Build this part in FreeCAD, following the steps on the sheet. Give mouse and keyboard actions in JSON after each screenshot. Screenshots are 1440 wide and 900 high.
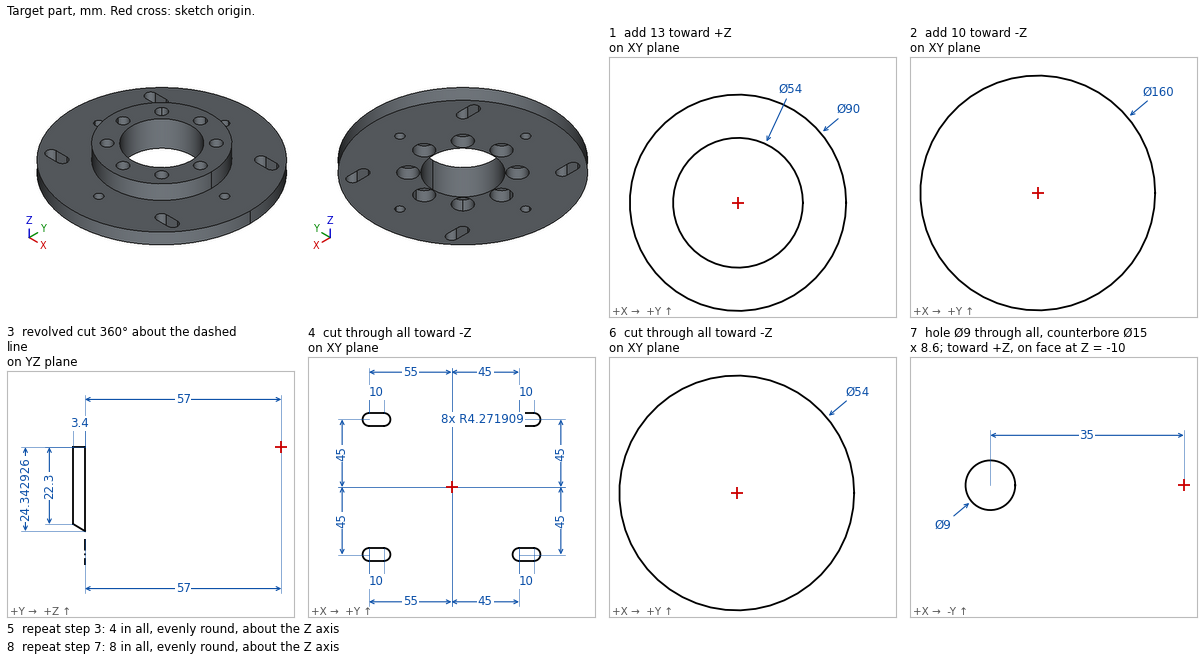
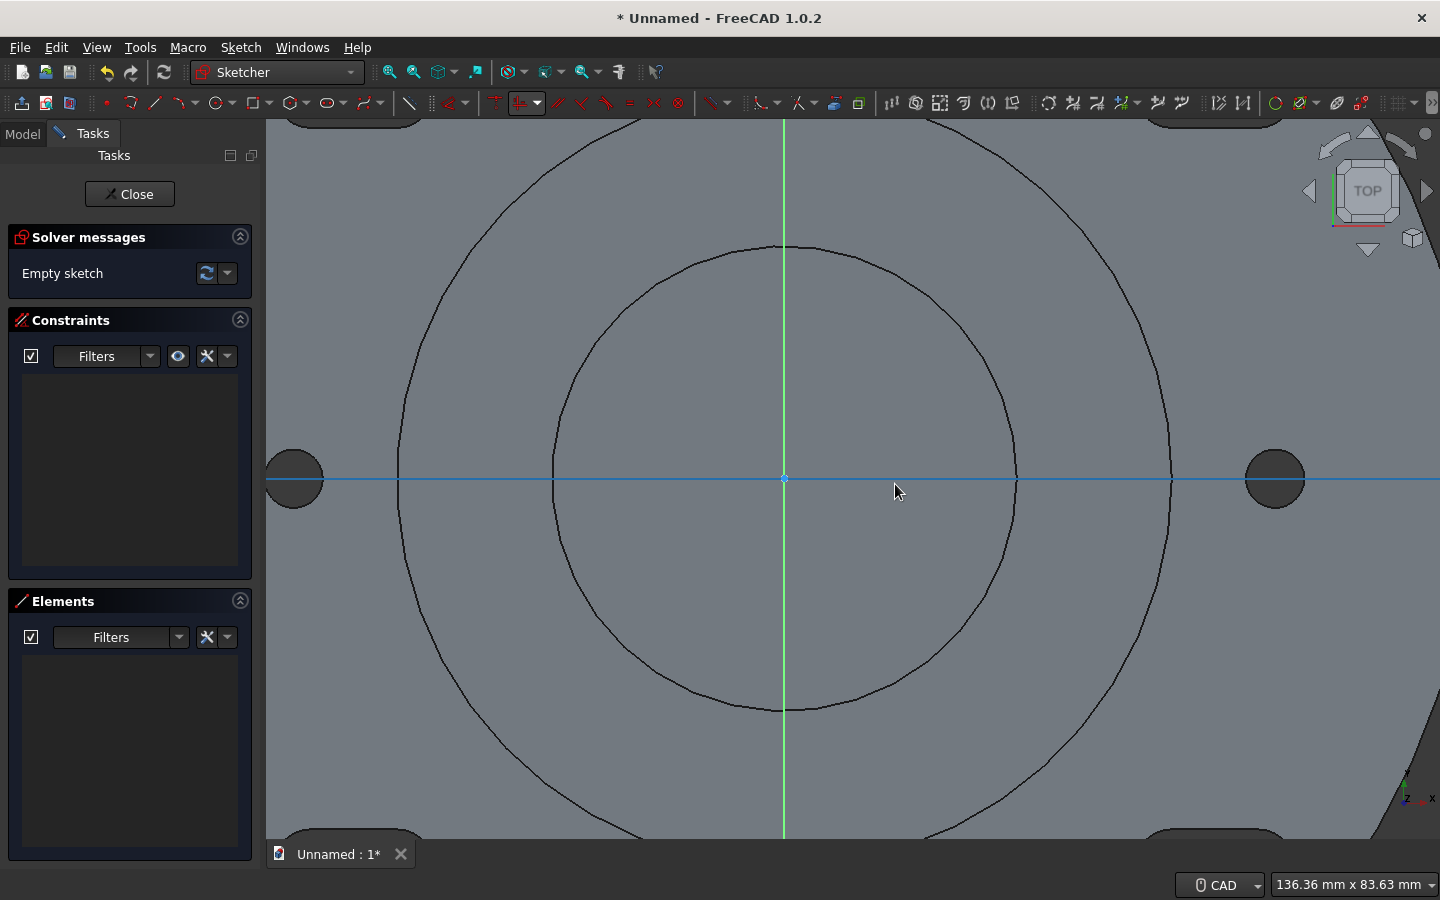
{"action": "key", "text": "g c"}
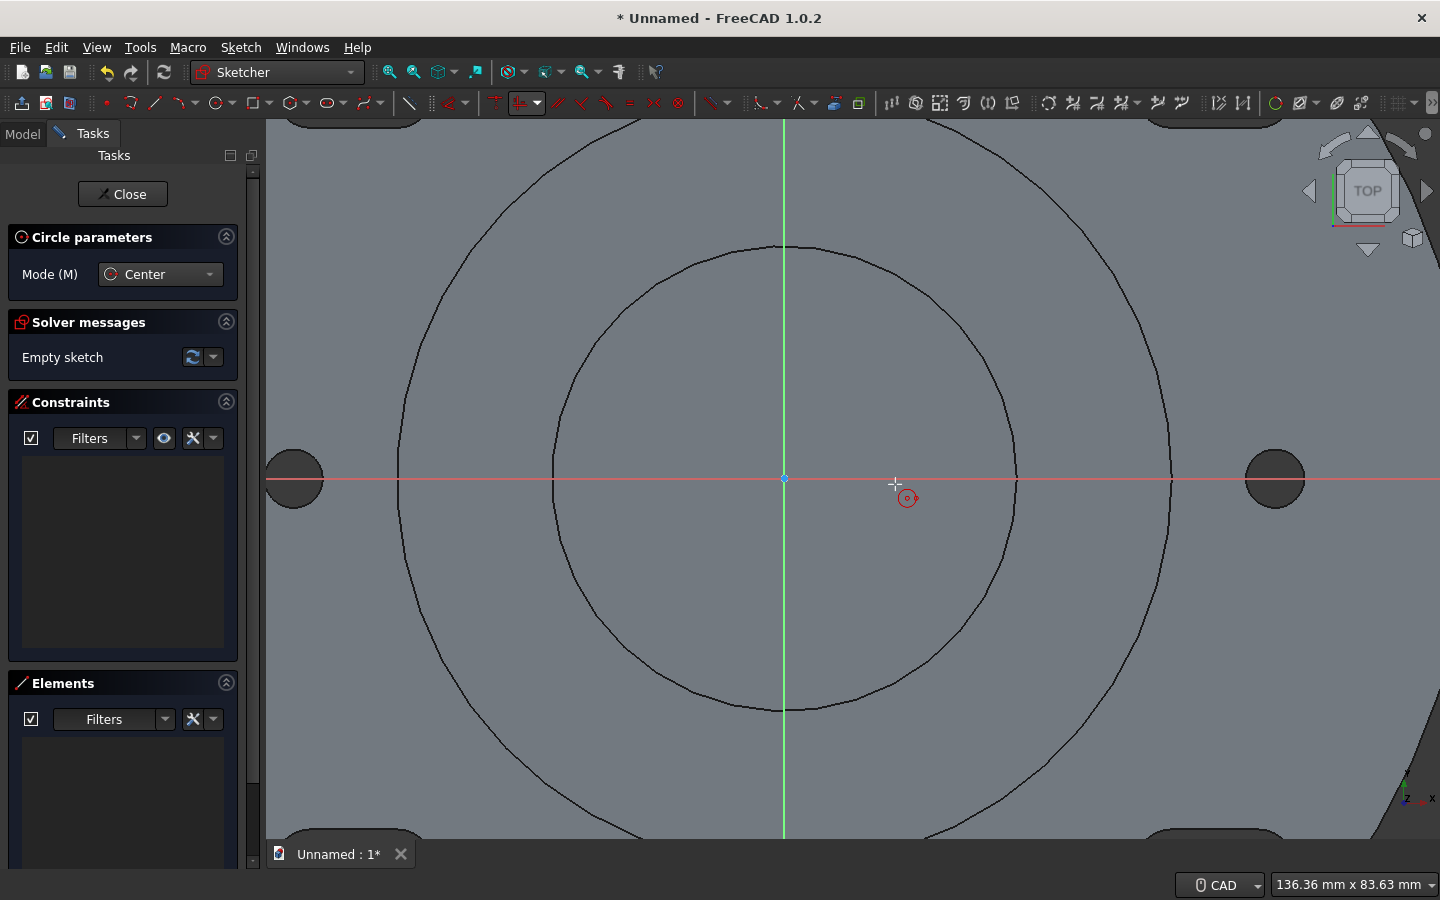
{"action": "left_click", "coordinate": [784, 479]}
{"action": "mouse_move", "coordinate": [949, 314]}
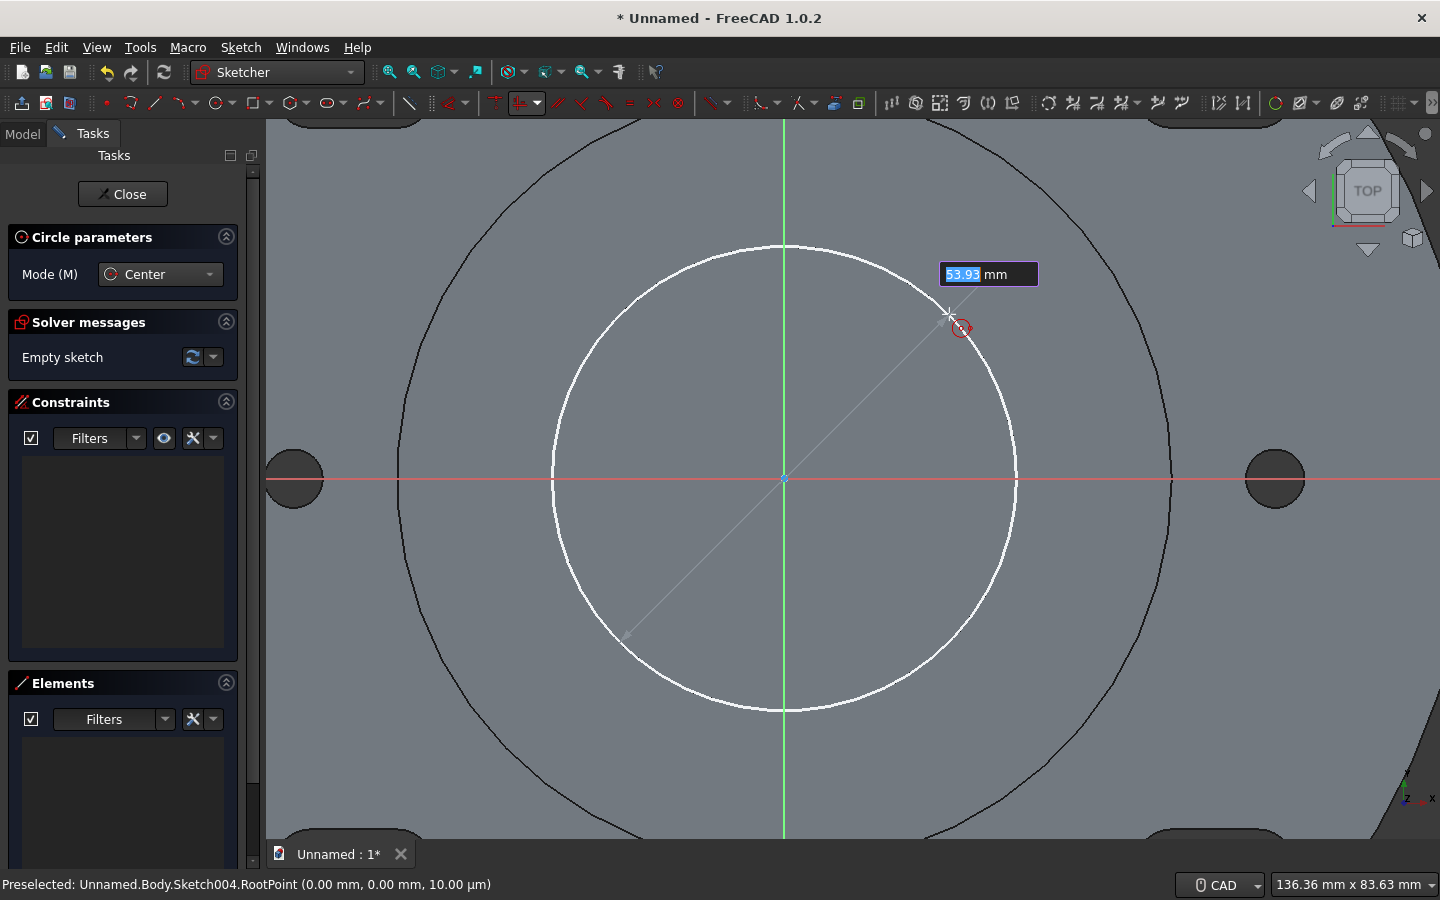
{"action": "type", "text": "54"}
{"action": "key", "text": "Return"}
{"action": "key", "text": "Escape"}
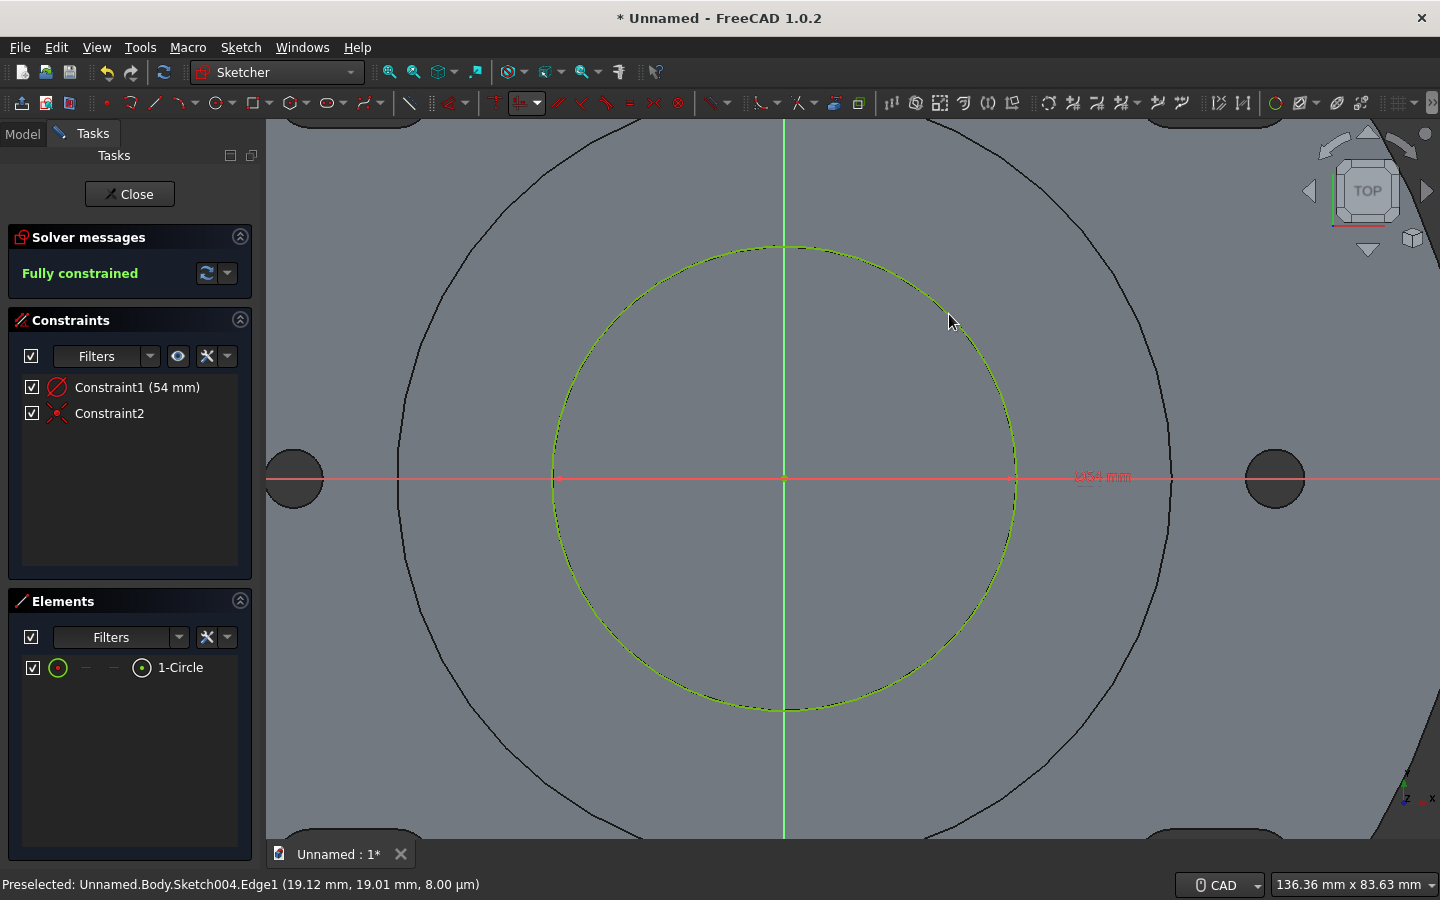
{"action": "left_click", "coordinate": [130, 194]}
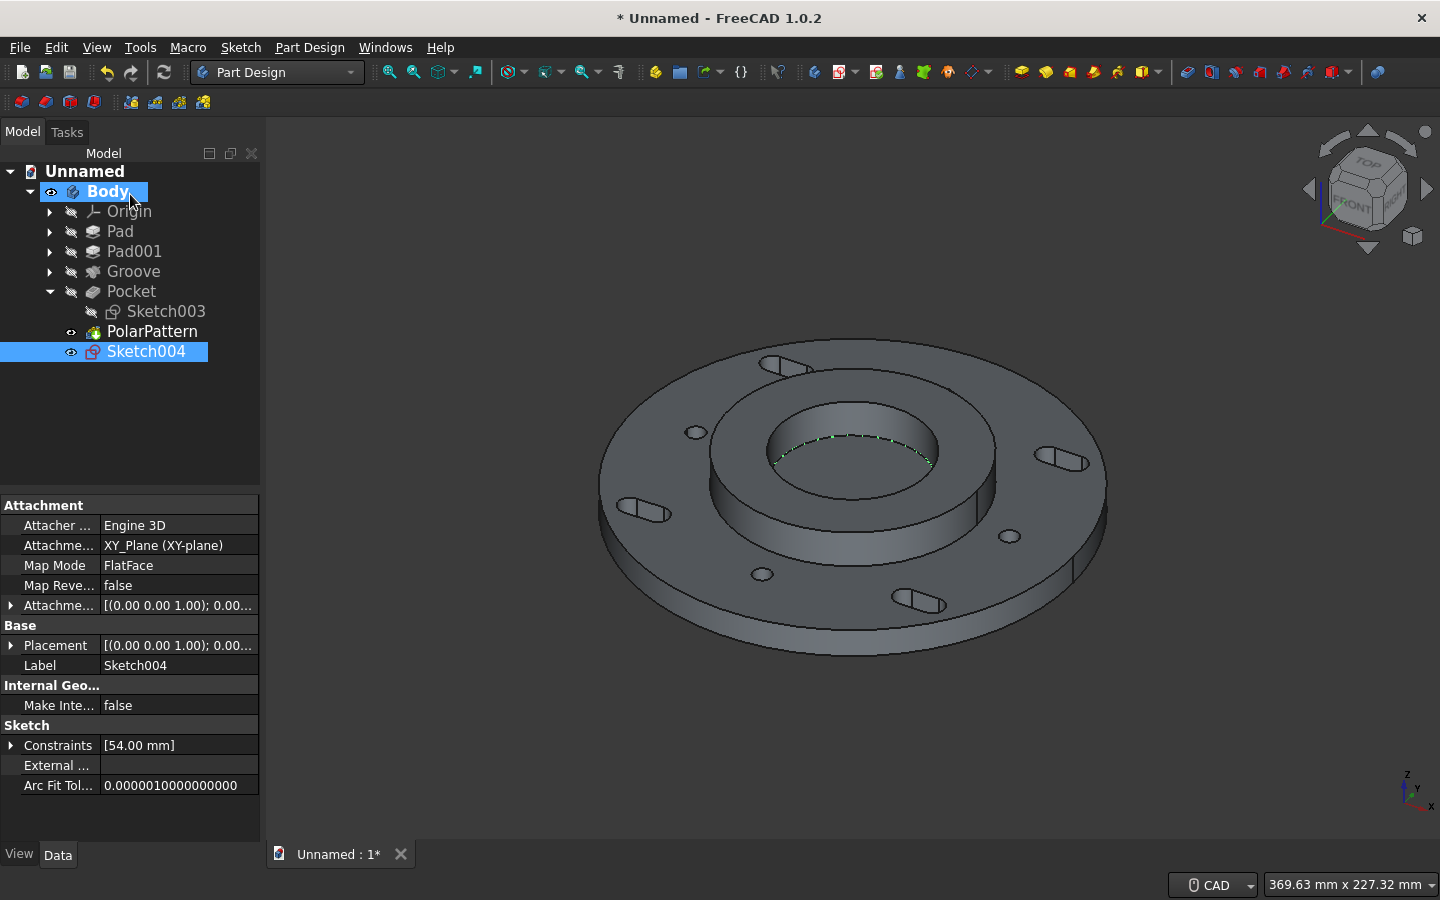
{"action": "left_click", "coordinate": [1188, 72]}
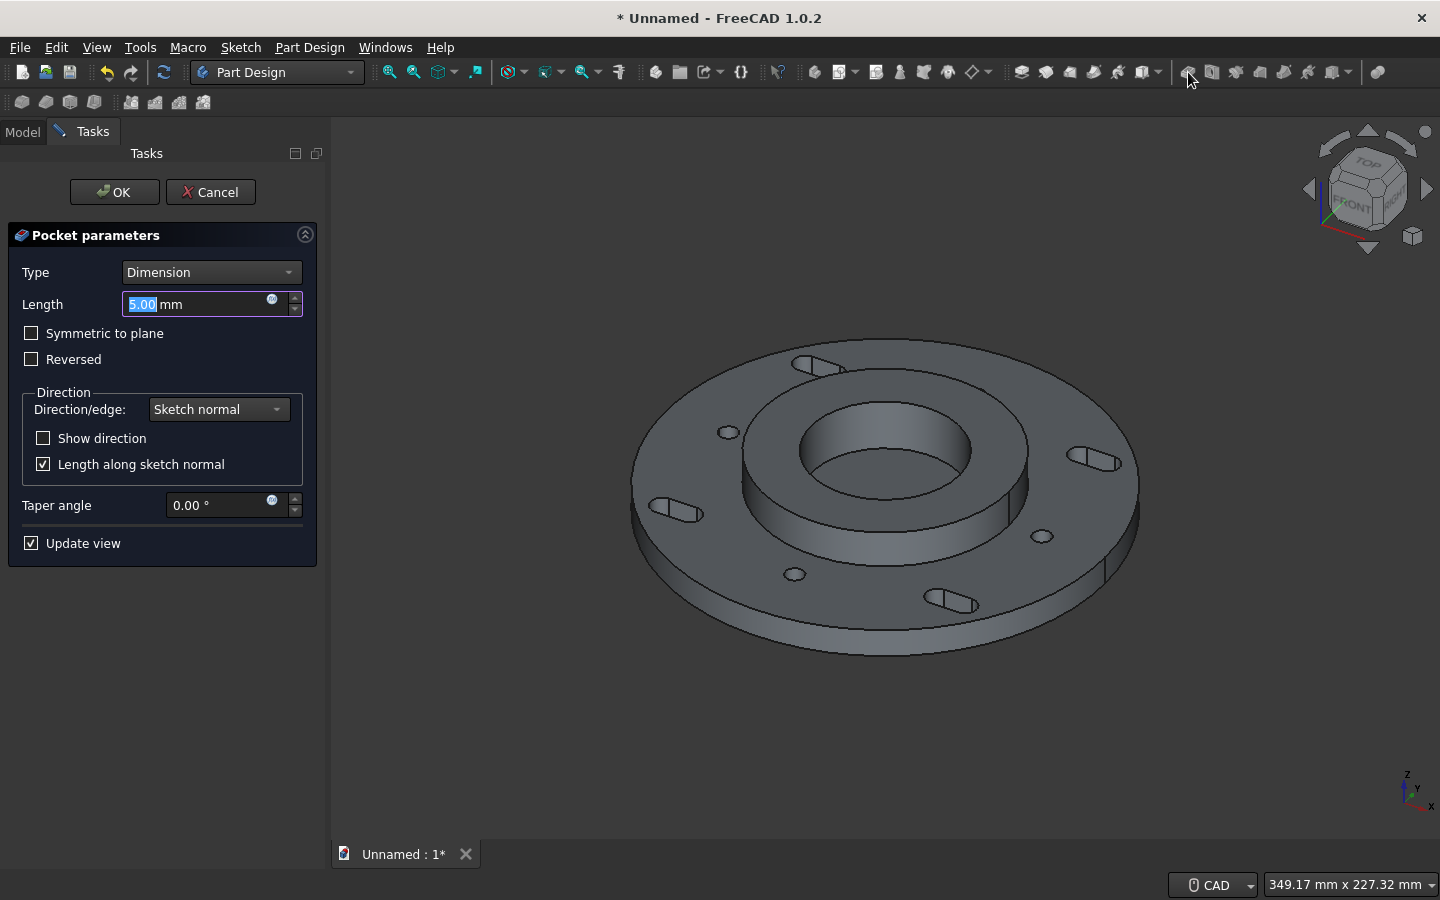
{"action": "left_click", "coordinate": [212, 272]}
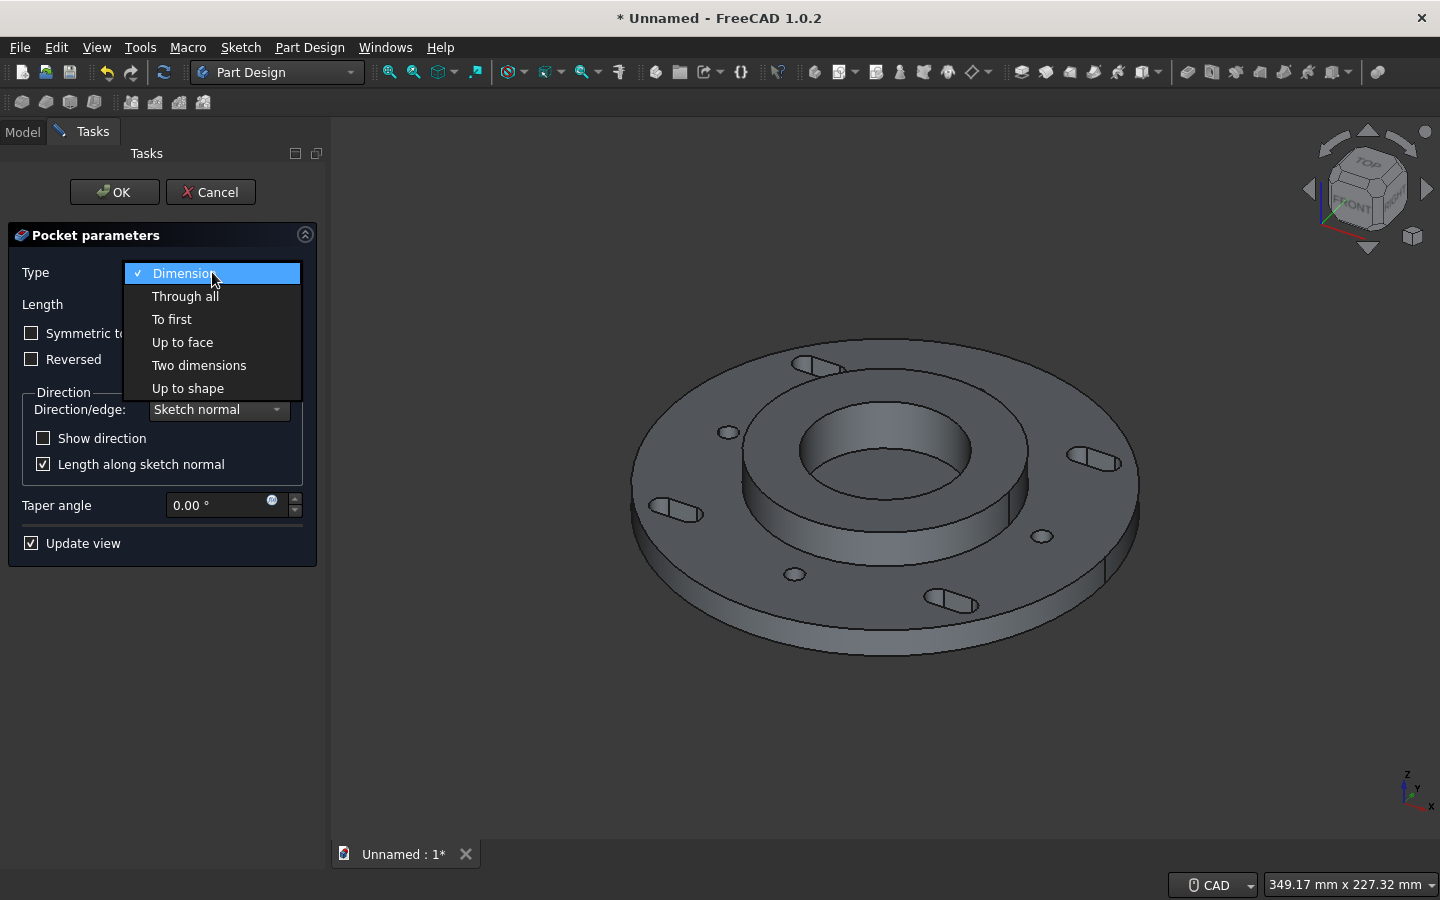
{"action": "left_click", "coordinate": [212, 296]}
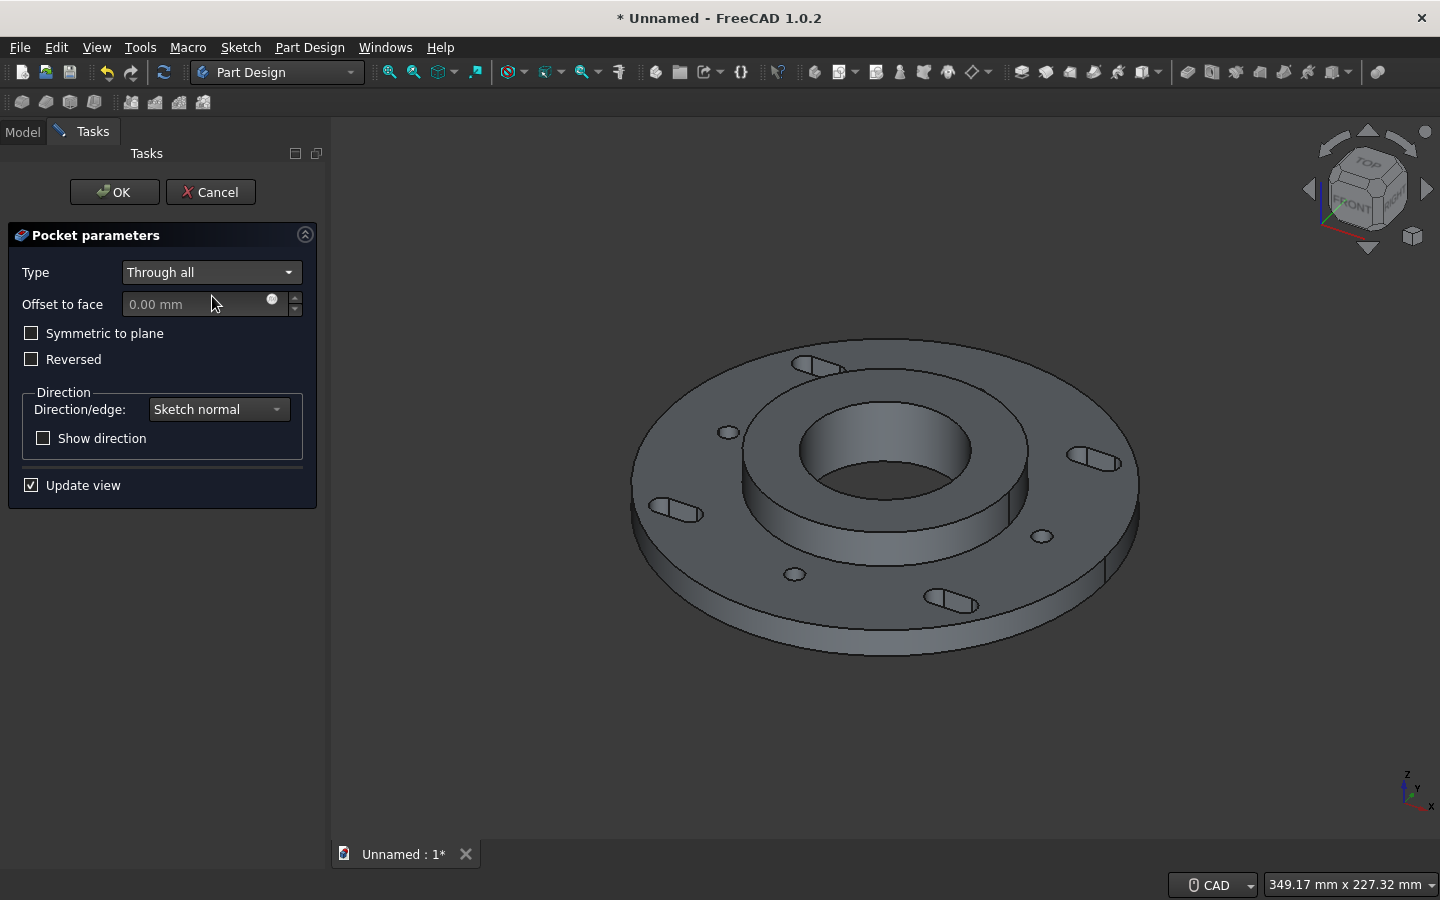
{"action": "left_click", "coordinate": [115, 192]}